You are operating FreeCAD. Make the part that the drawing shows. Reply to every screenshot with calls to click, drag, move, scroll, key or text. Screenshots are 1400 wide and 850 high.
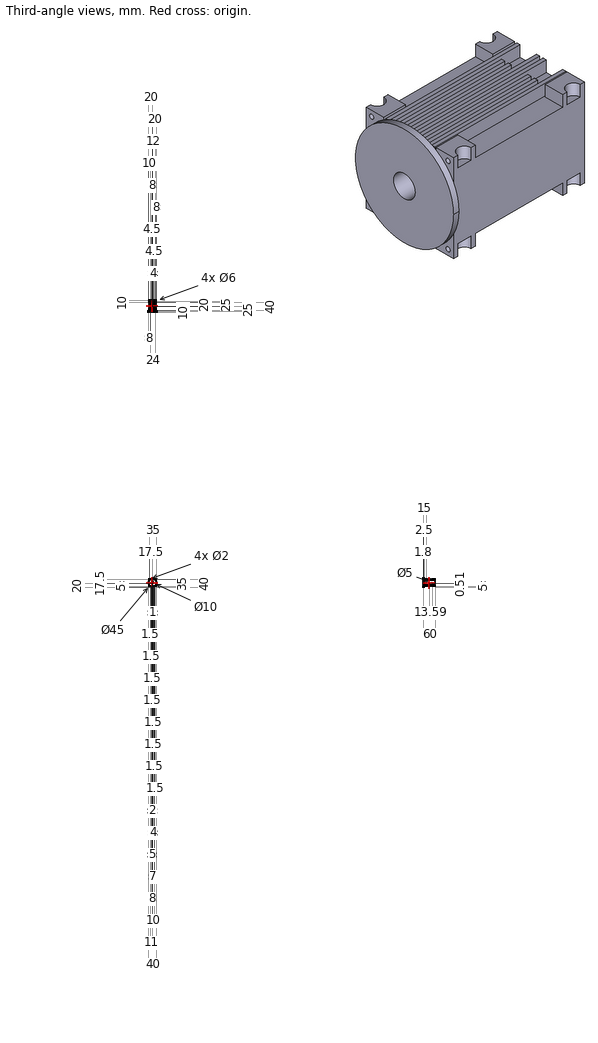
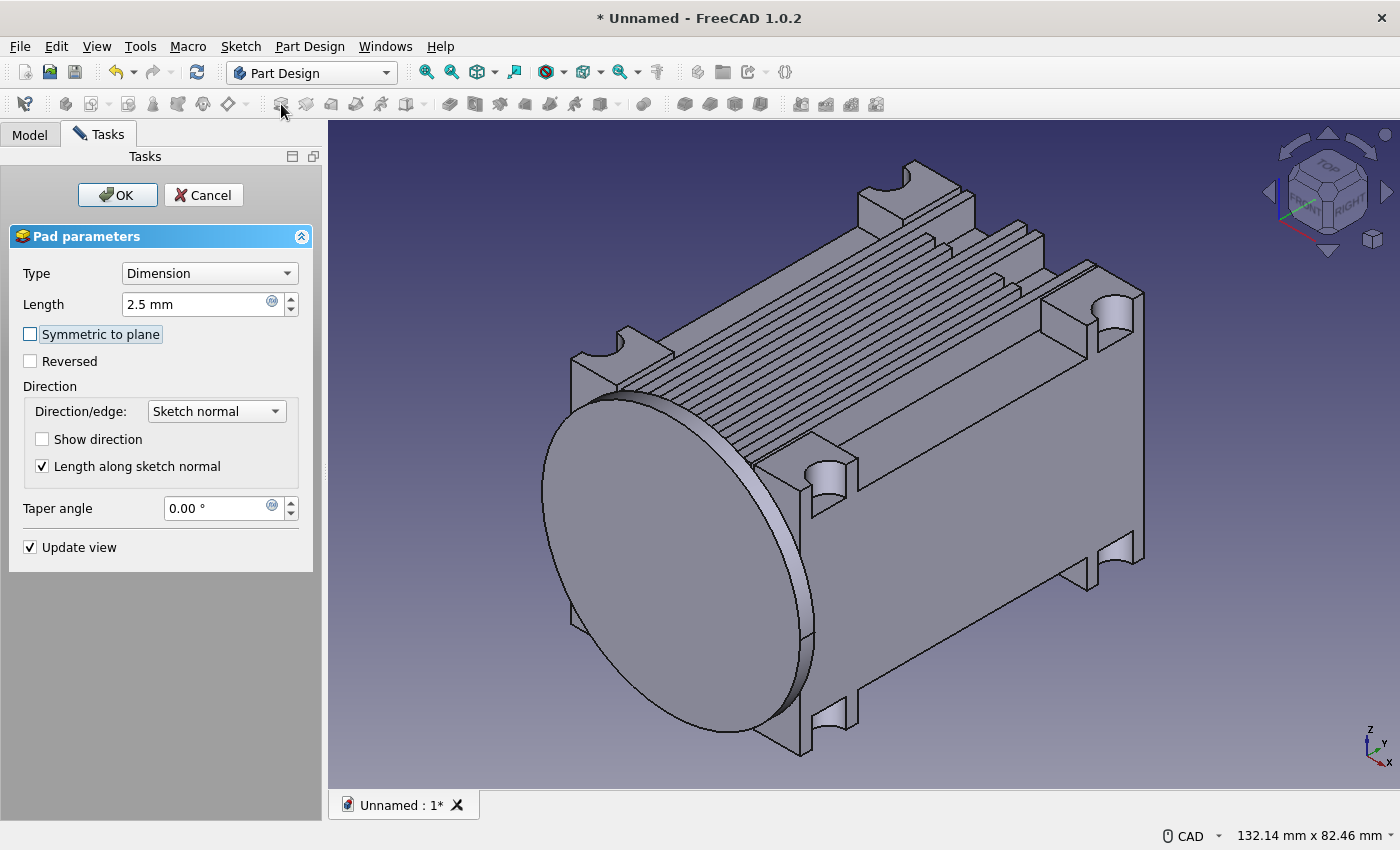
click(118, 195)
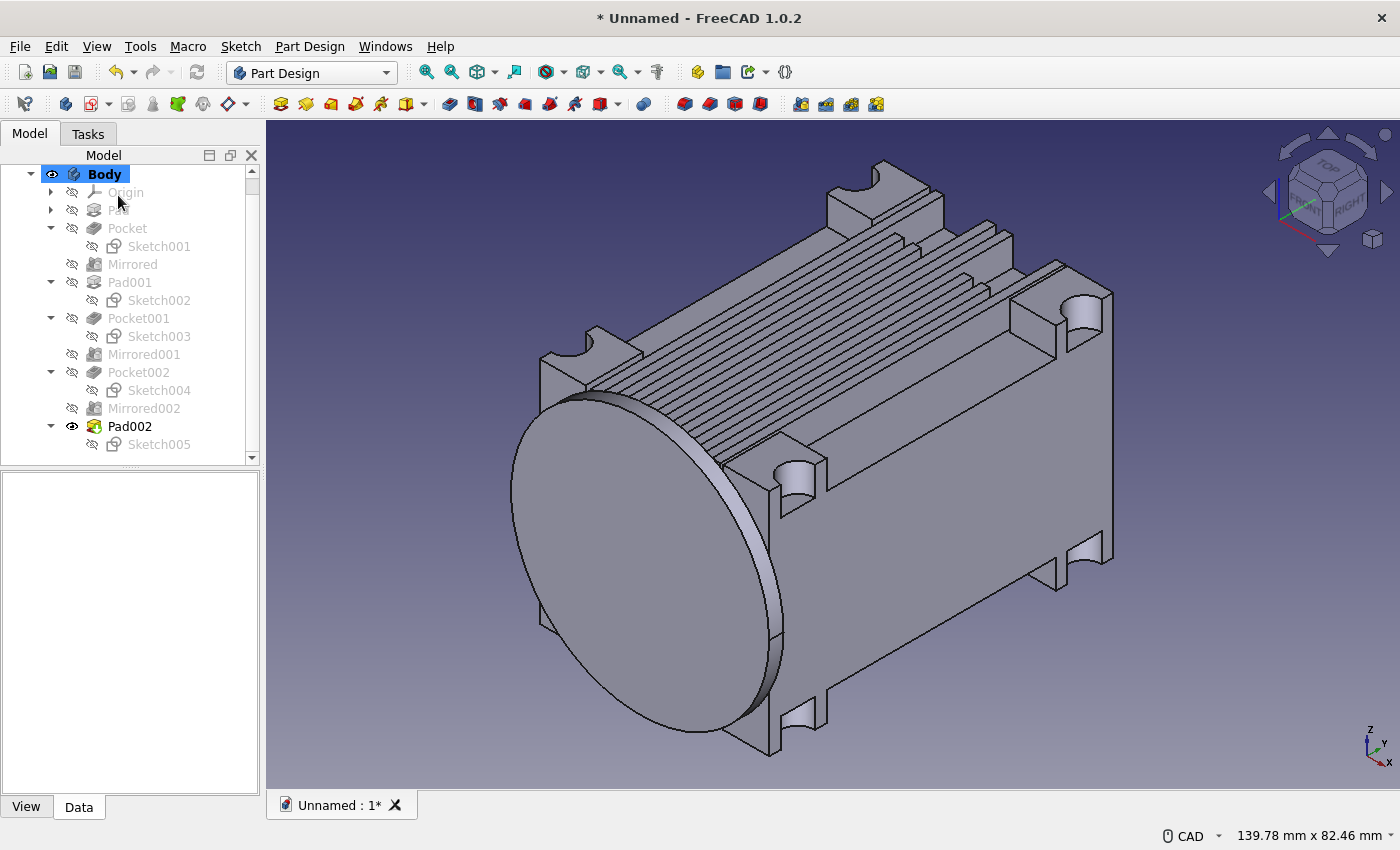
click(640, 565)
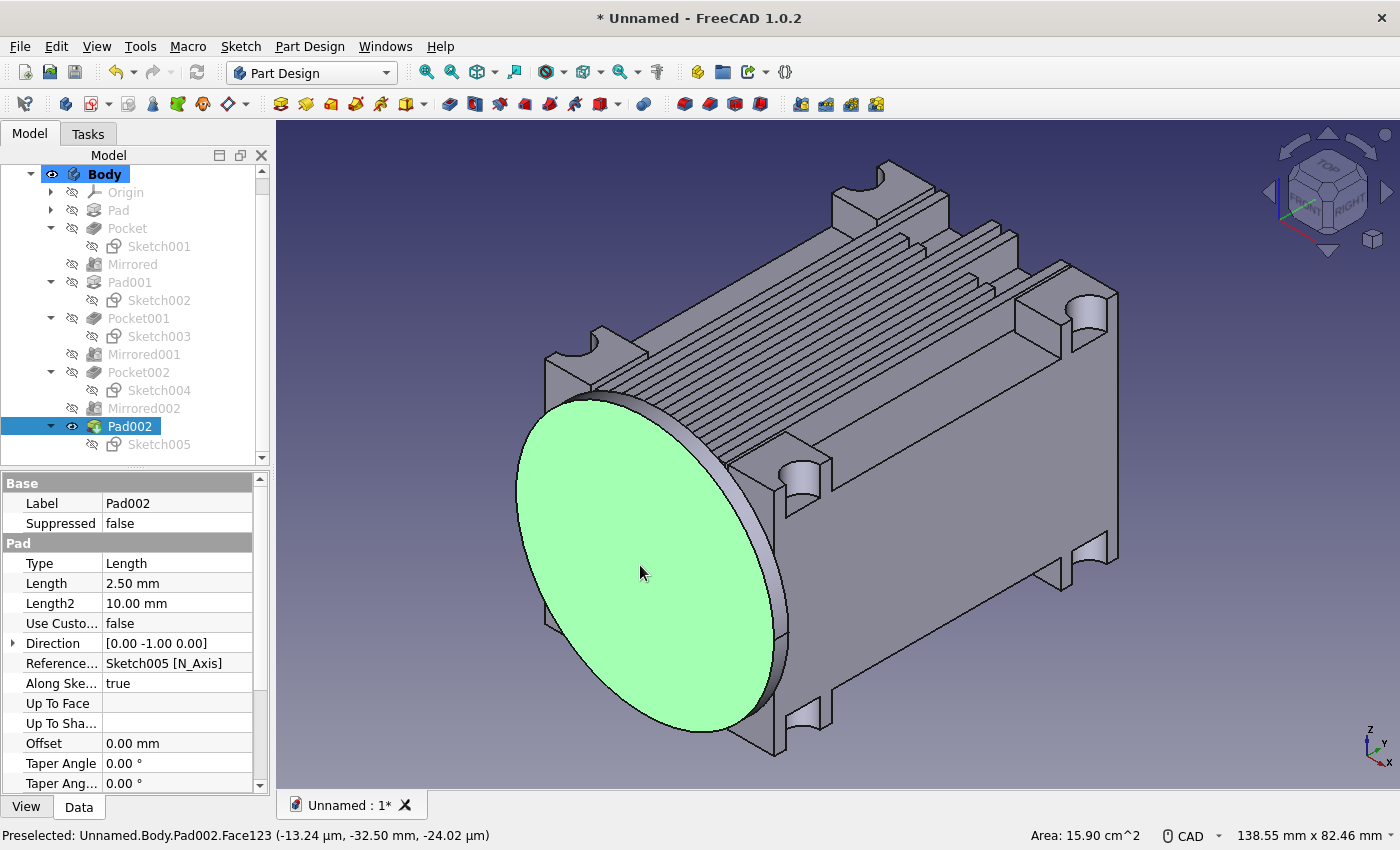
click(90, 104)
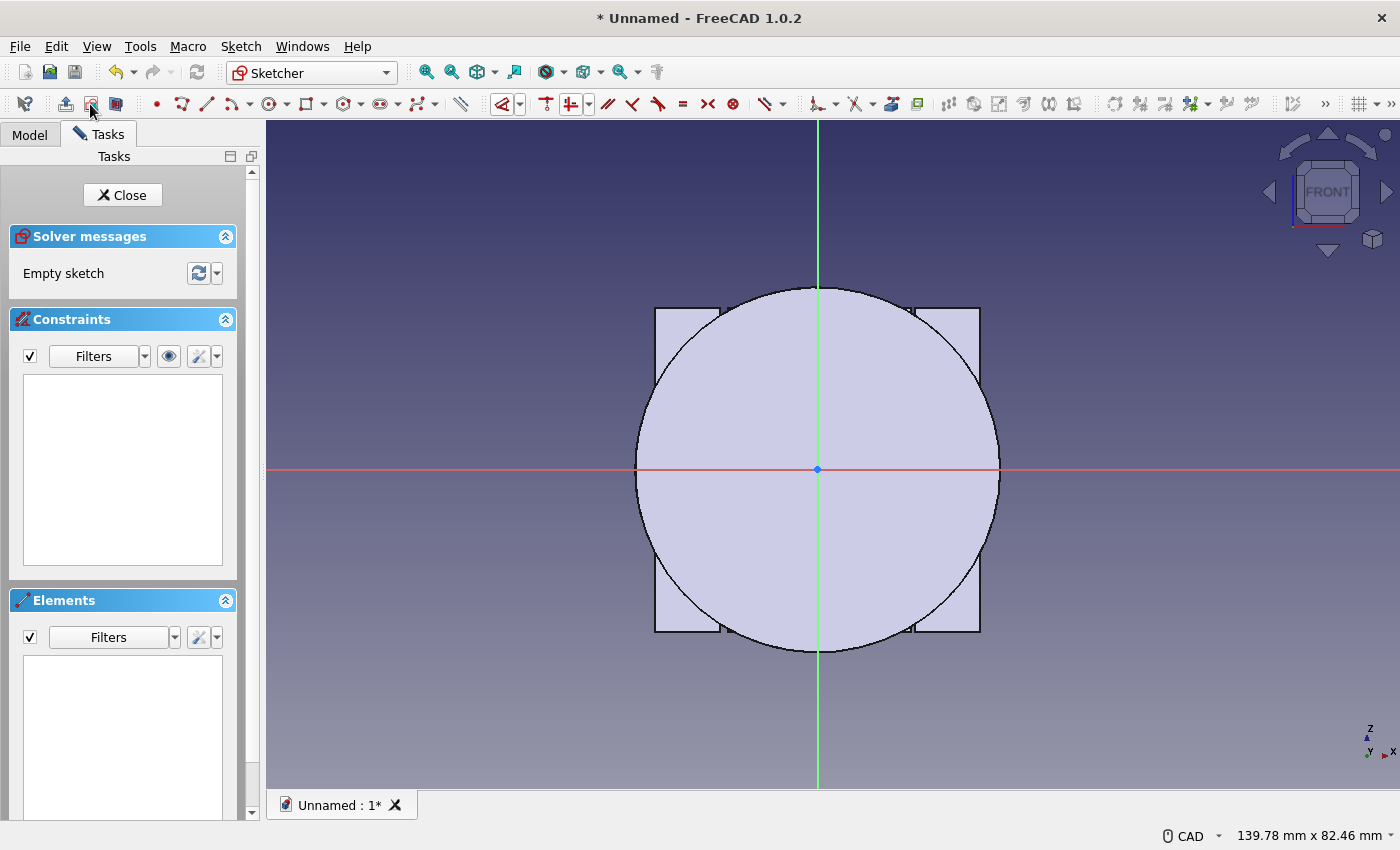
scroll(831, 474, up, 8)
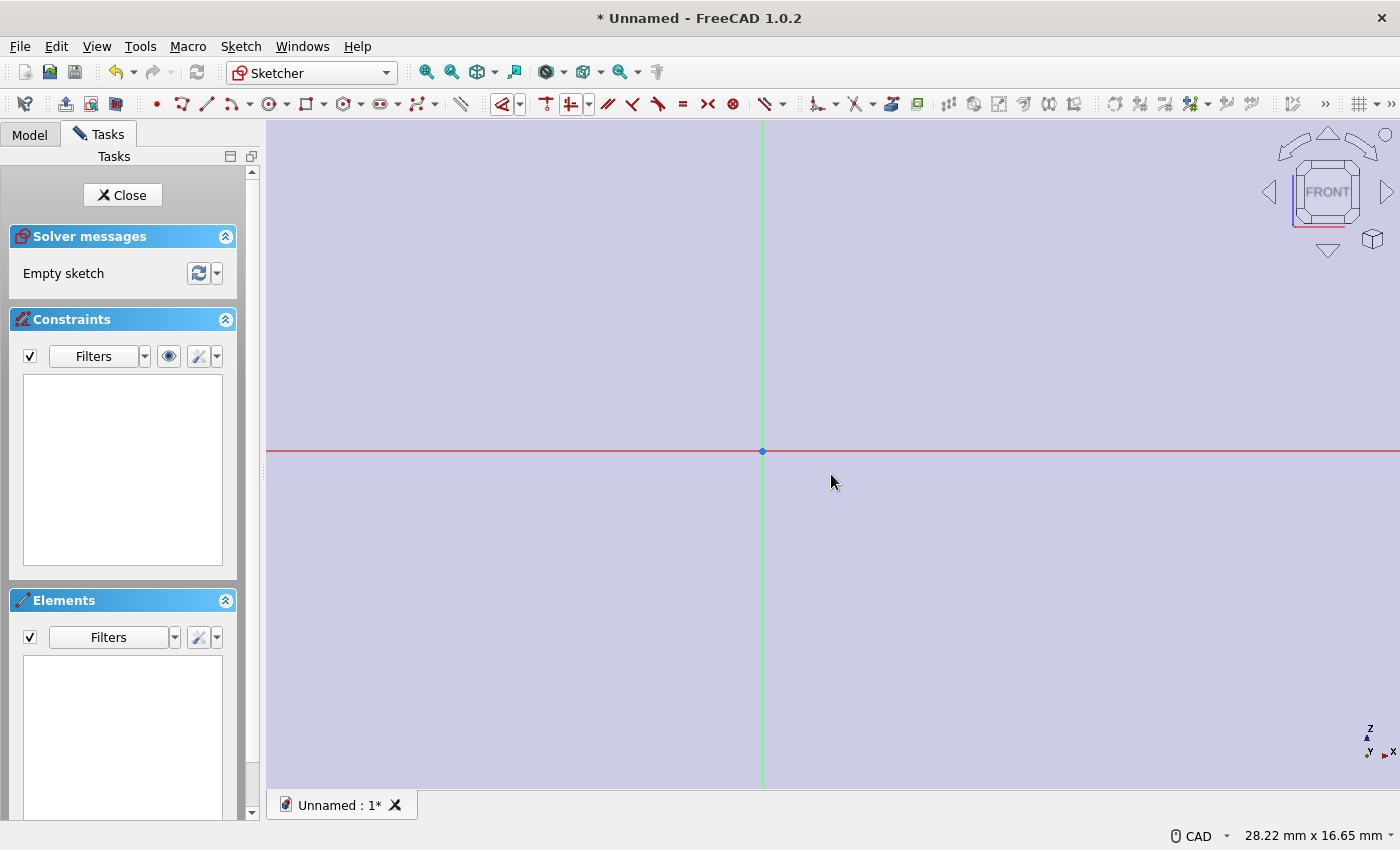
key(g)
key(c)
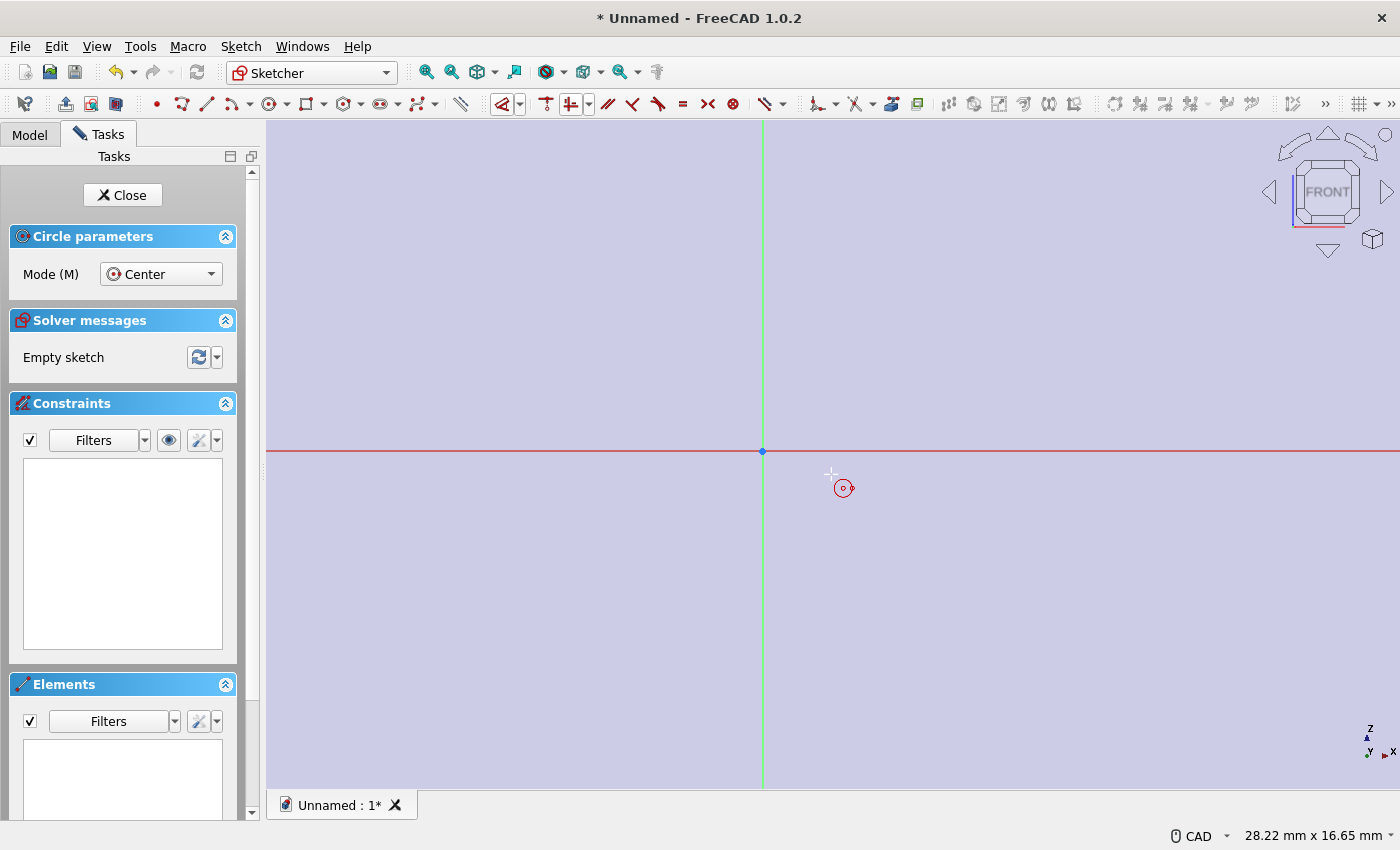
click(763, 451)
click(905, 309)
key(Escape)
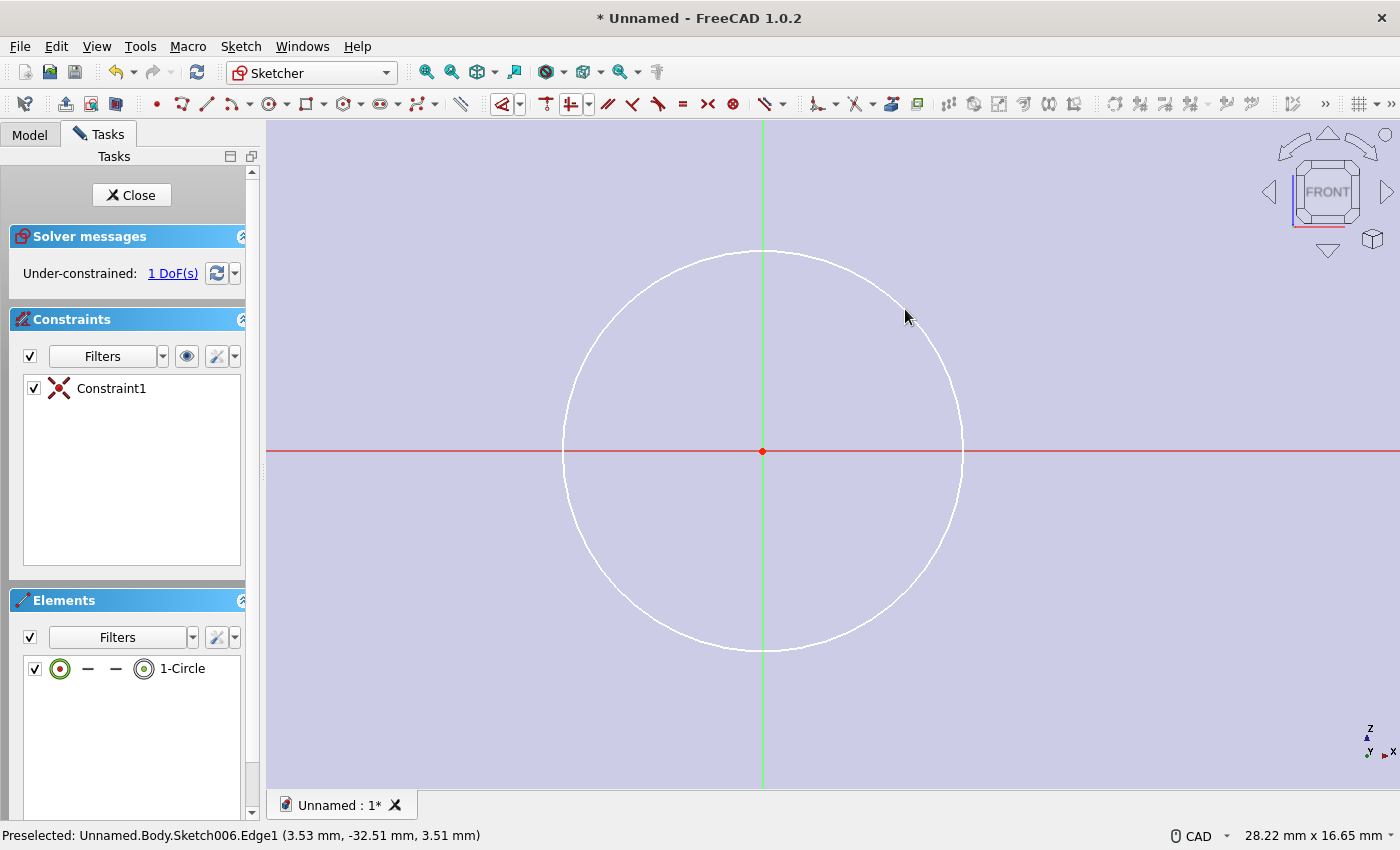
click(904, 309)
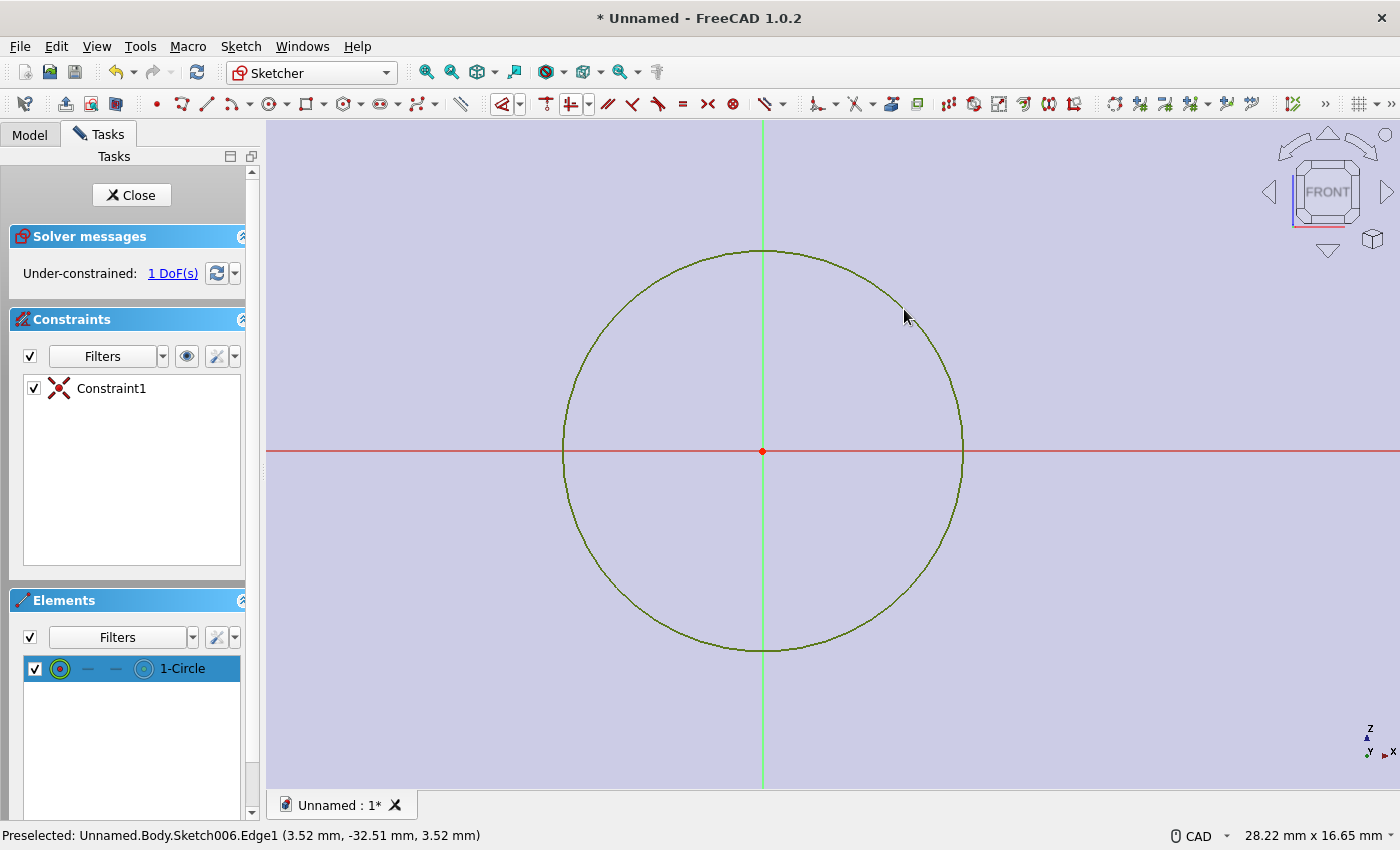
key(k)
key(o)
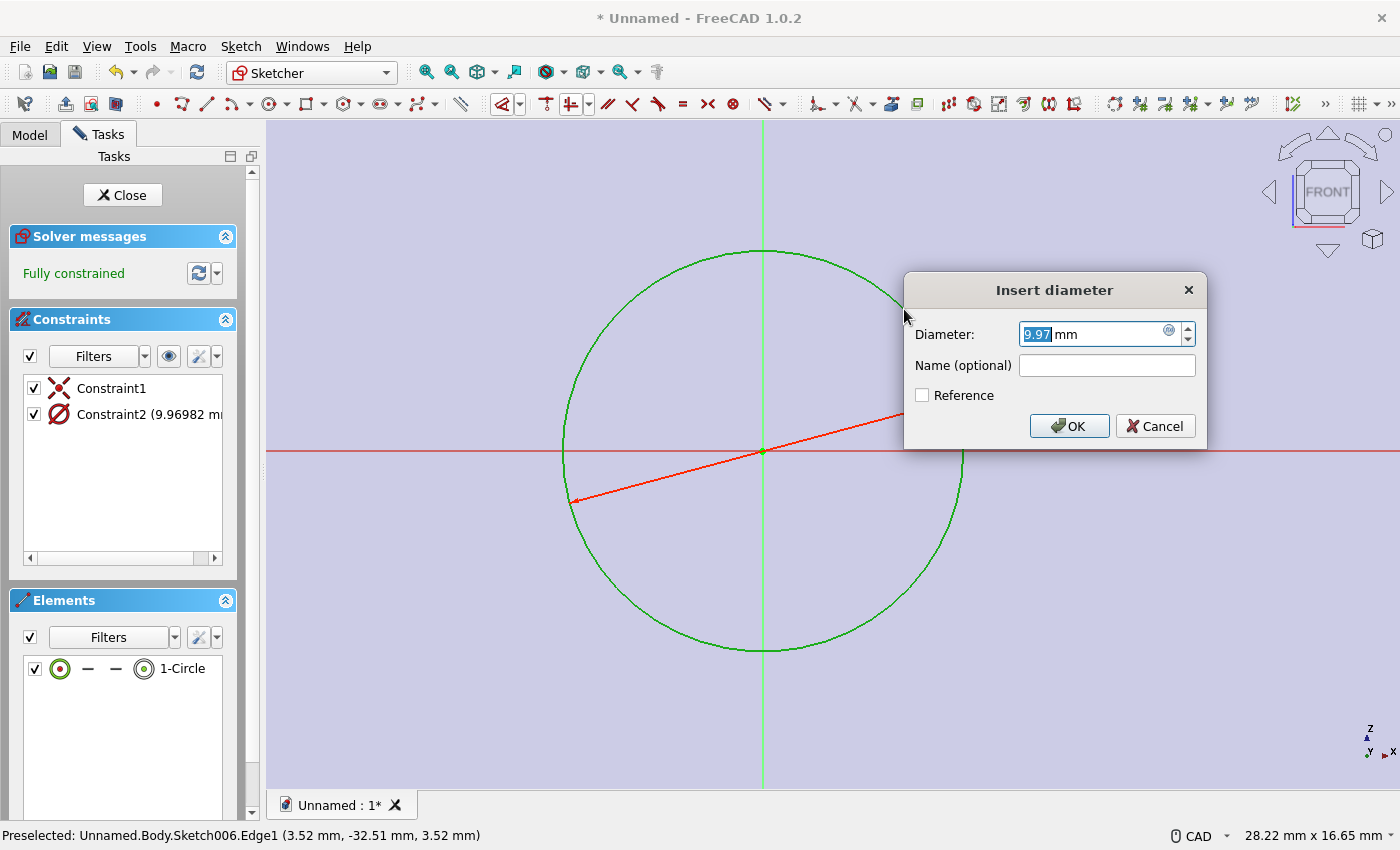
text(10)
key(Return)